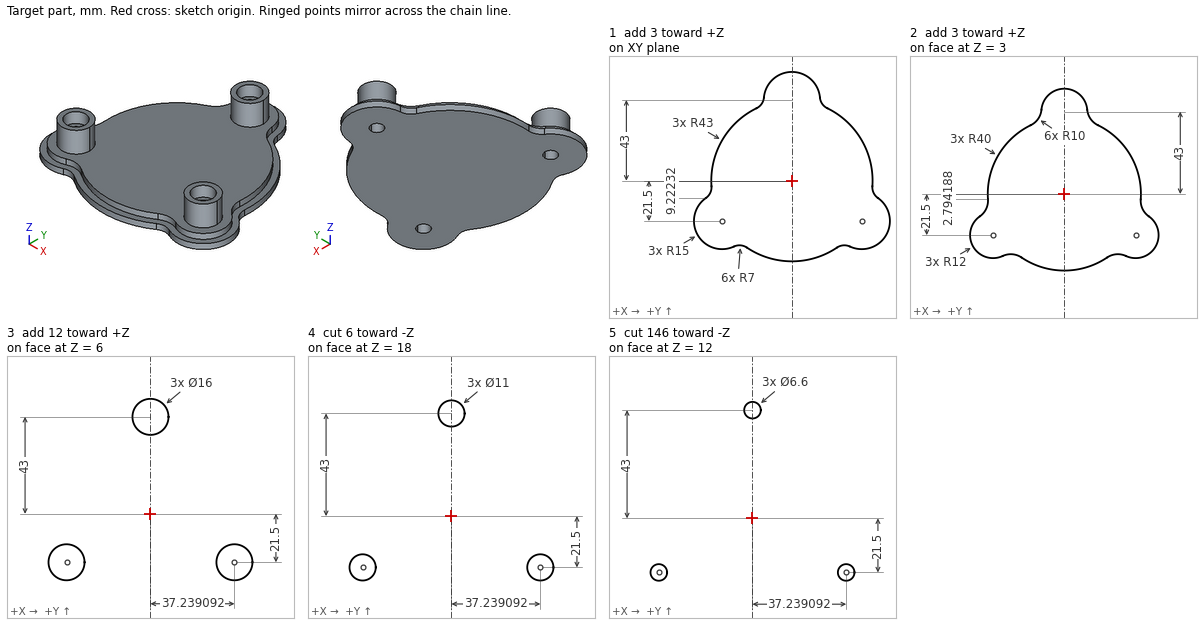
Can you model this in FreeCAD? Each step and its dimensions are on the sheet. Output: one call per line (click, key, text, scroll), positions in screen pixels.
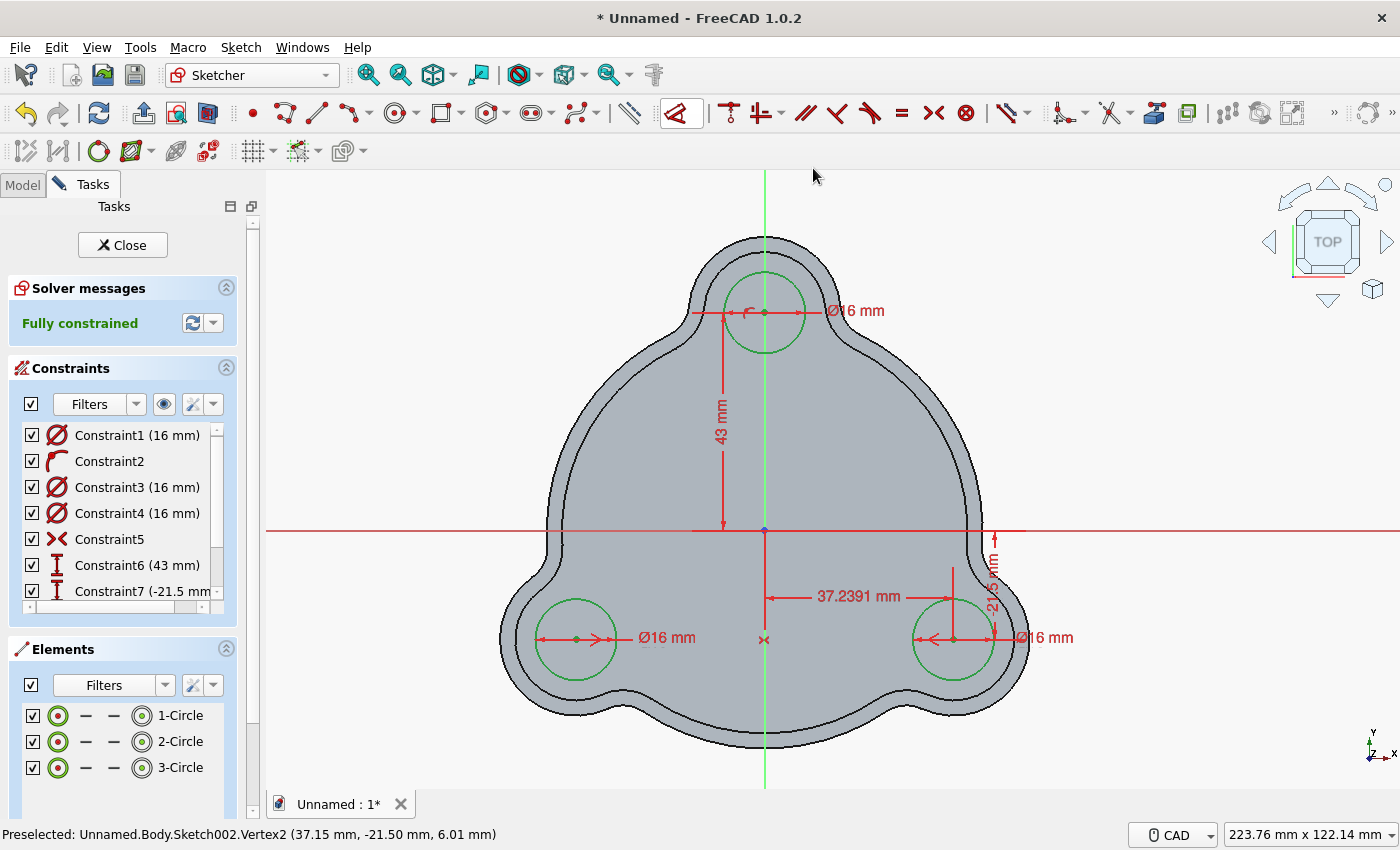
click(123, 245)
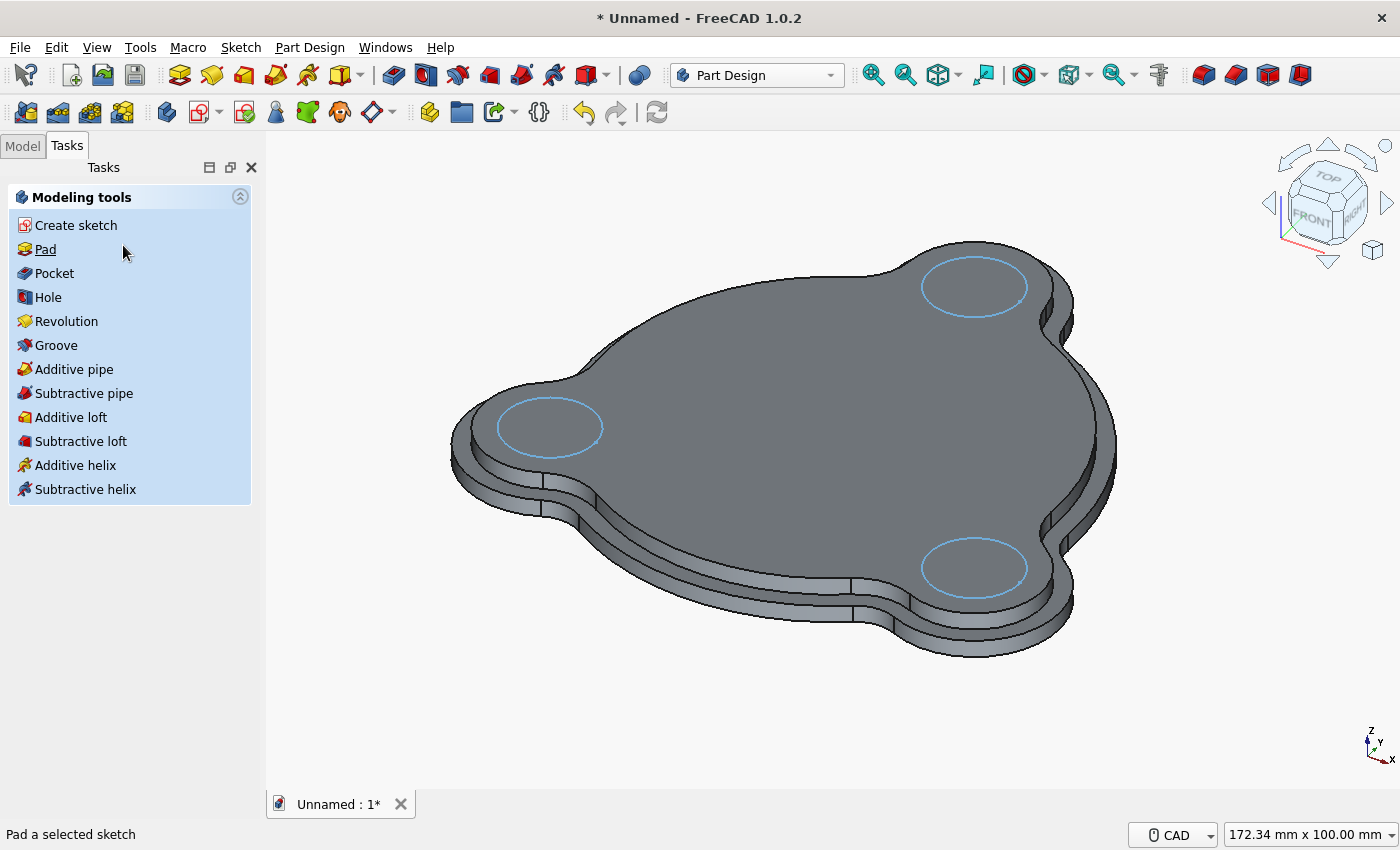
click(180, 76)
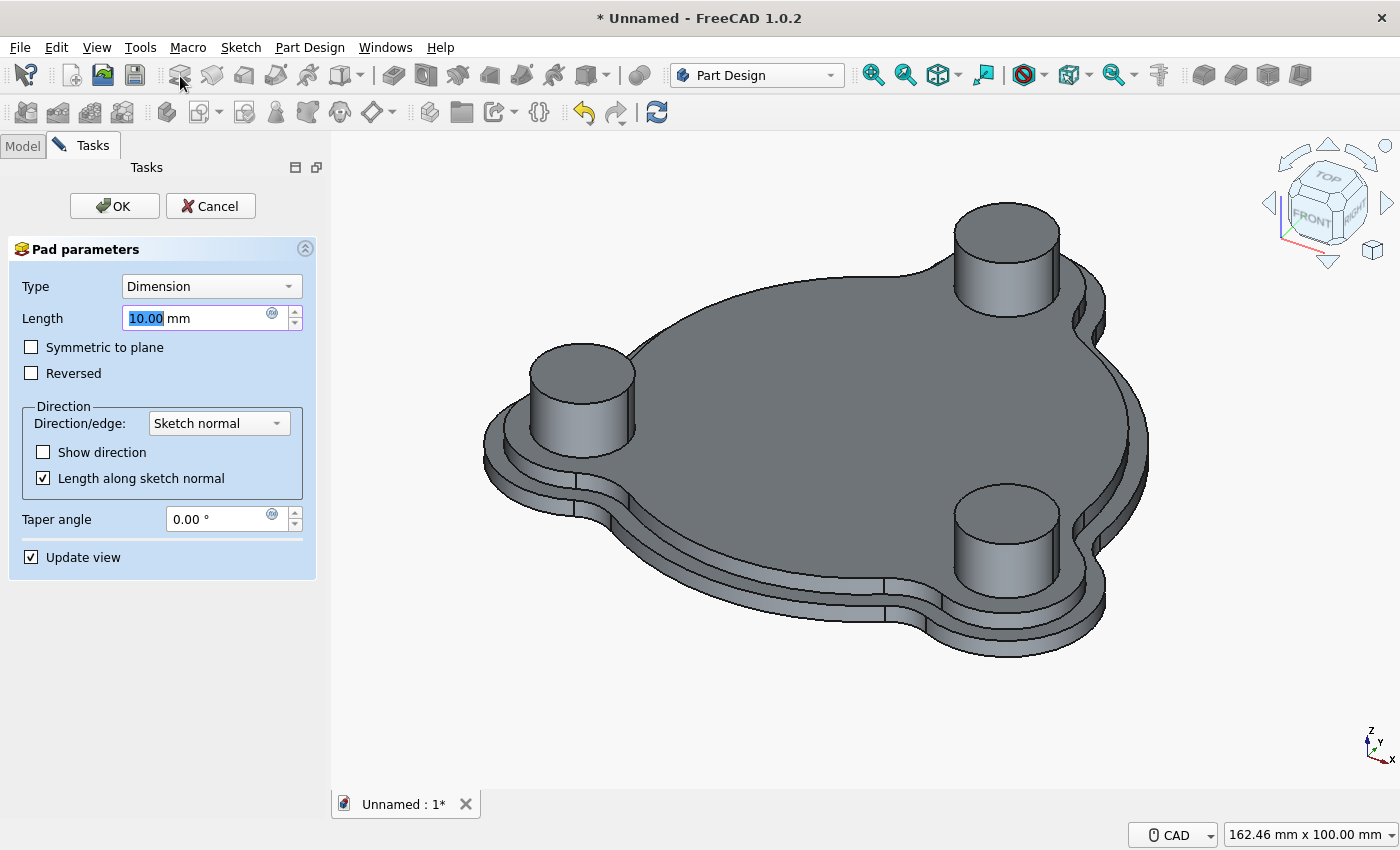
text(12)
key(Tab)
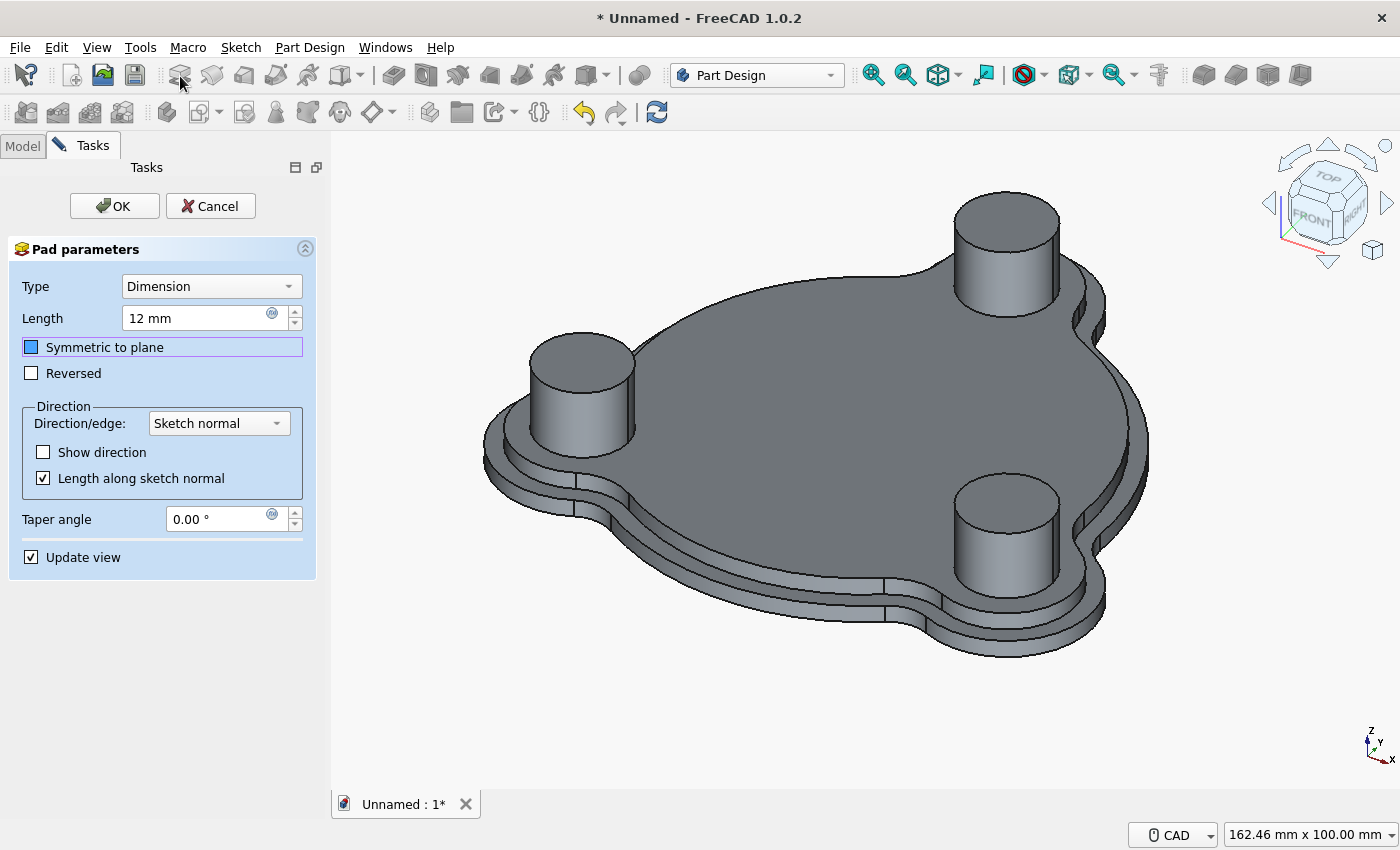
click(115, 206)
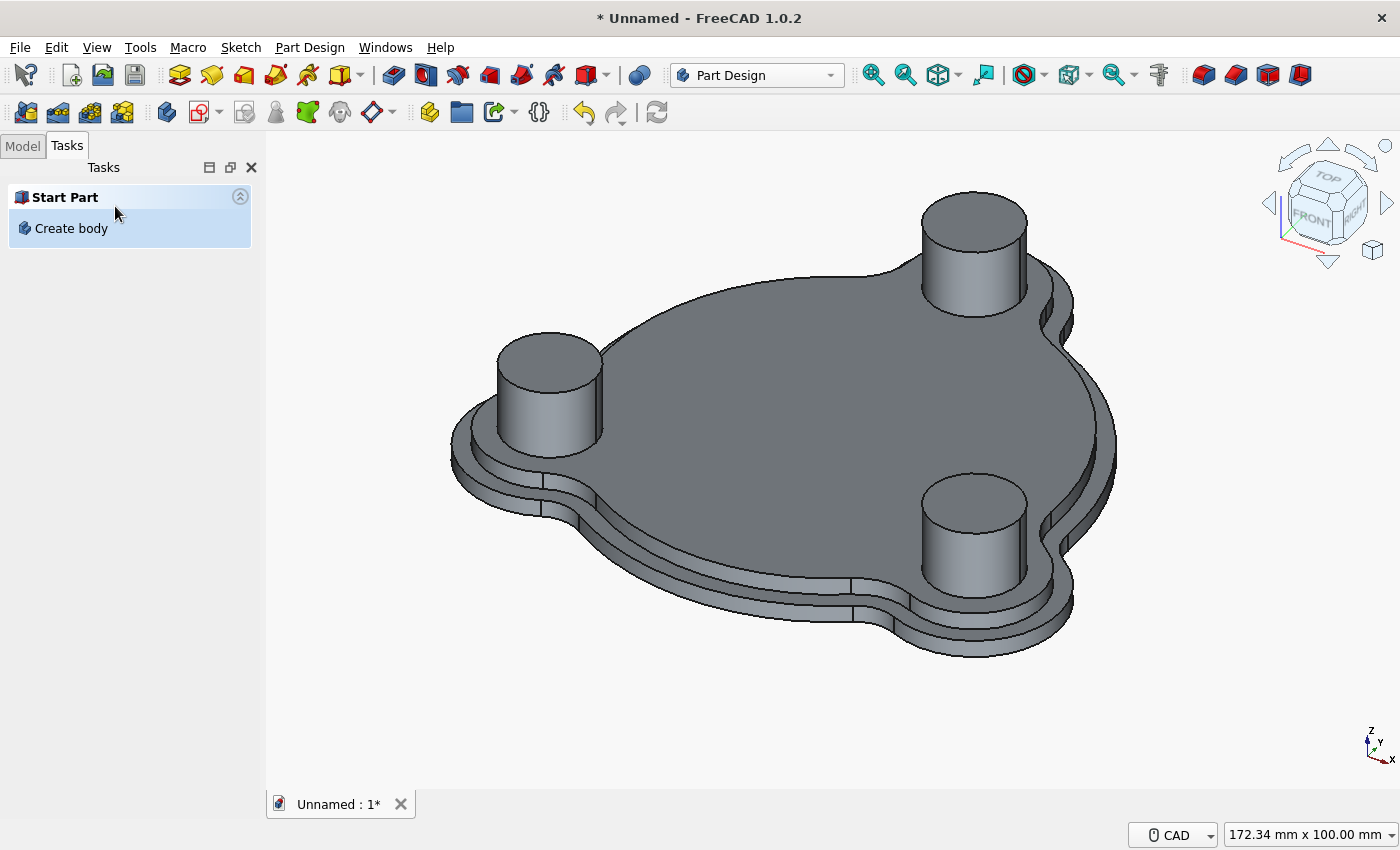
click(874, 76)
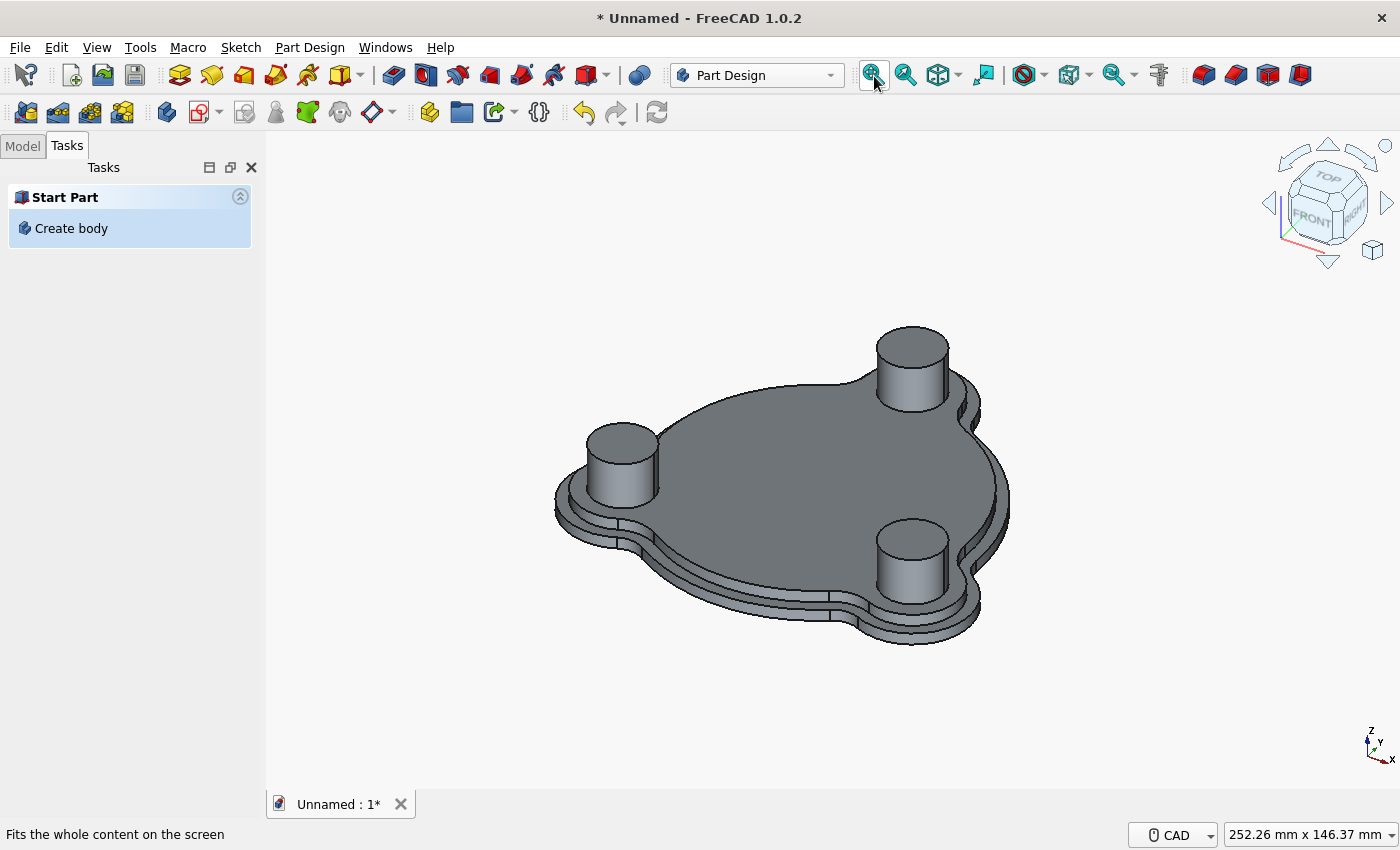
click(913, 539)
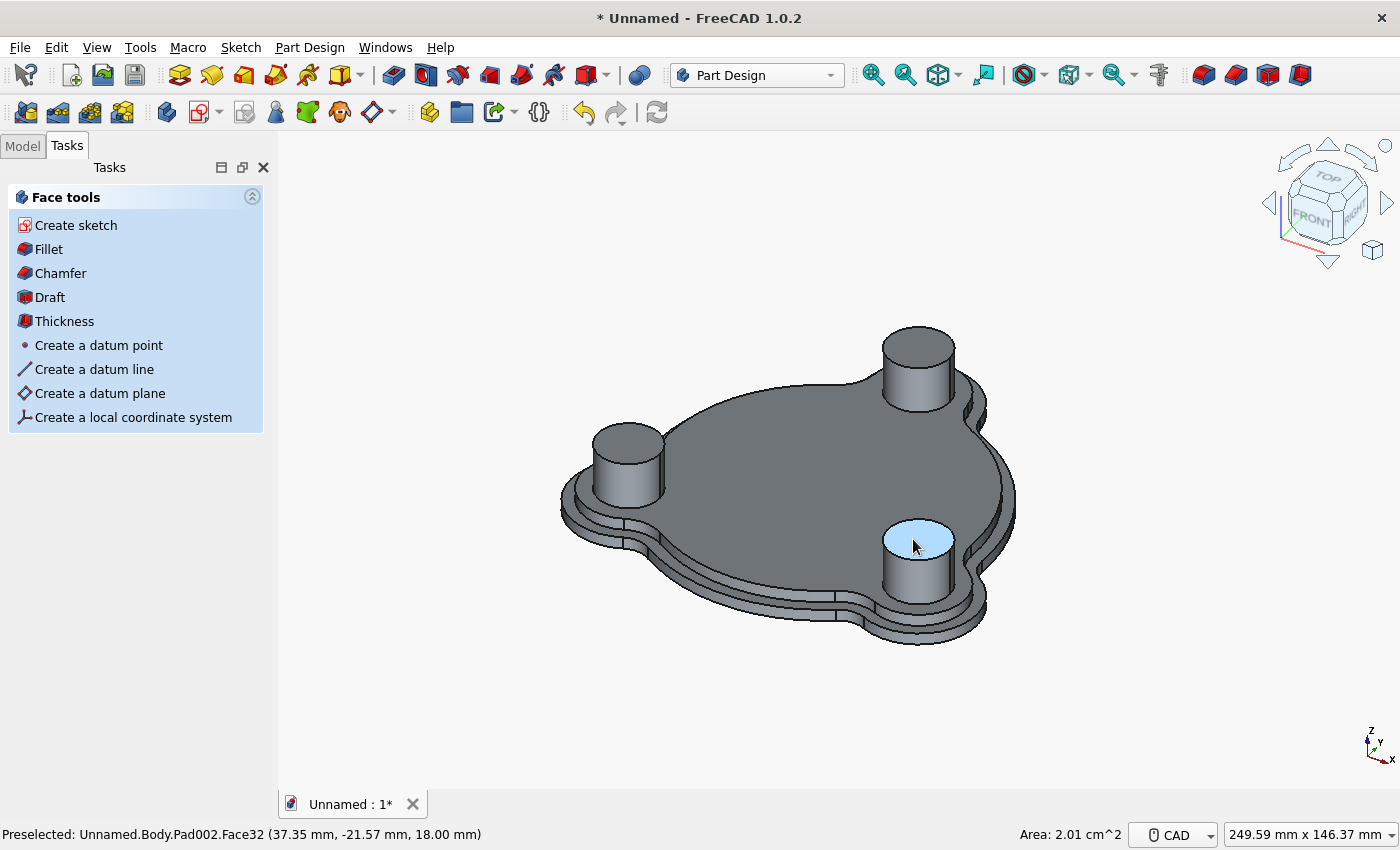
click(200, 112)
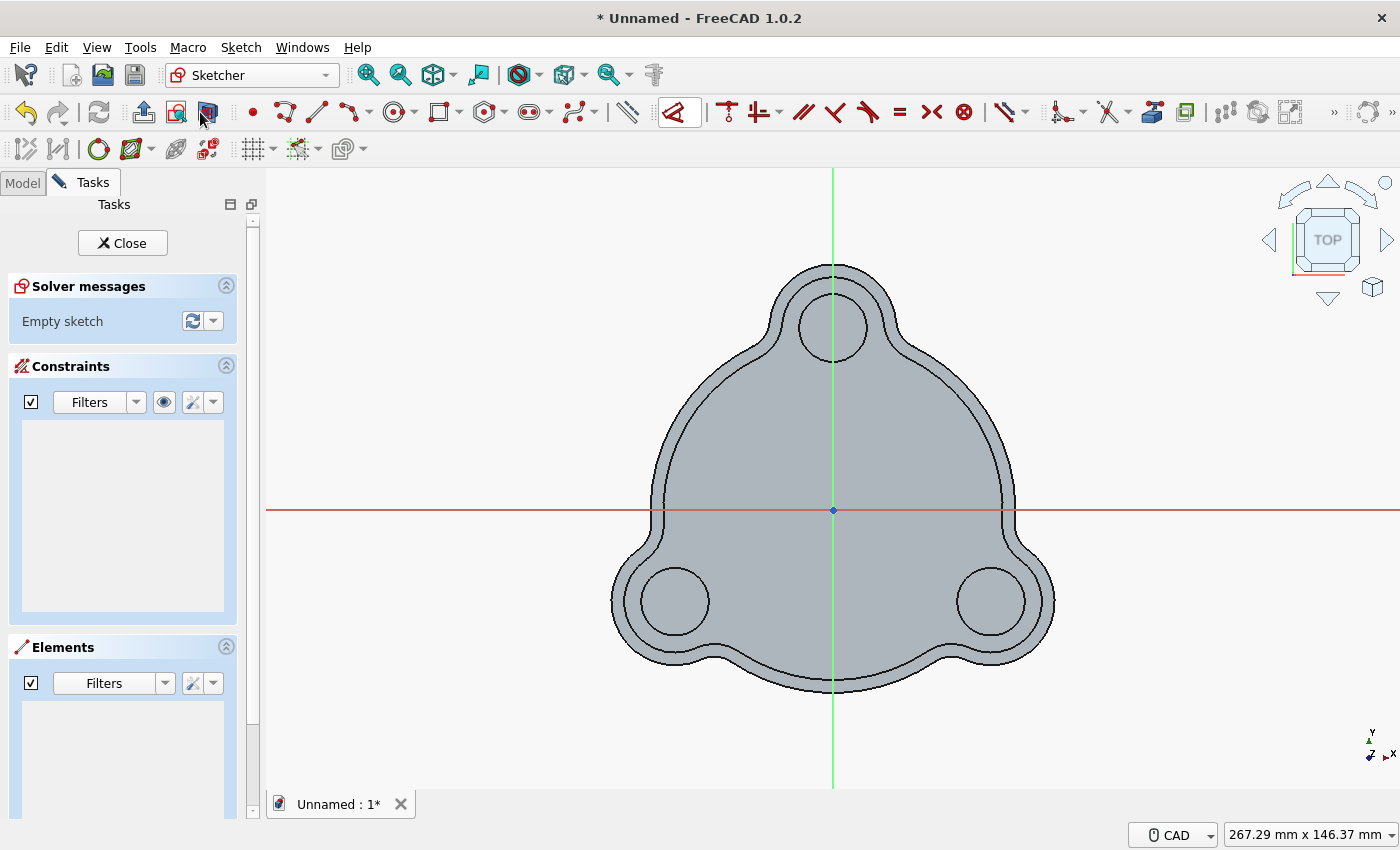
click(394, 112)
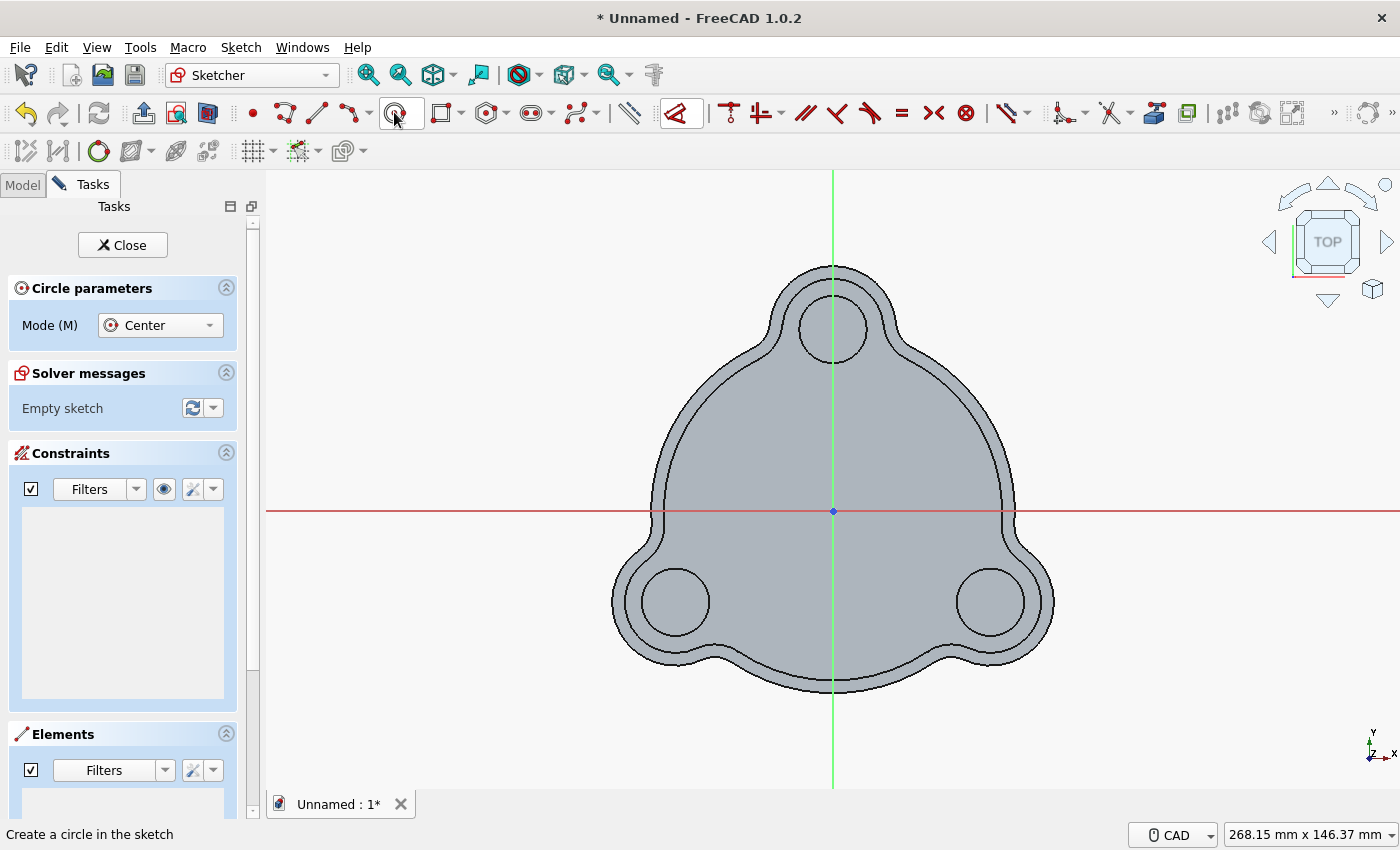
click(833, 330)
move(849, 313)